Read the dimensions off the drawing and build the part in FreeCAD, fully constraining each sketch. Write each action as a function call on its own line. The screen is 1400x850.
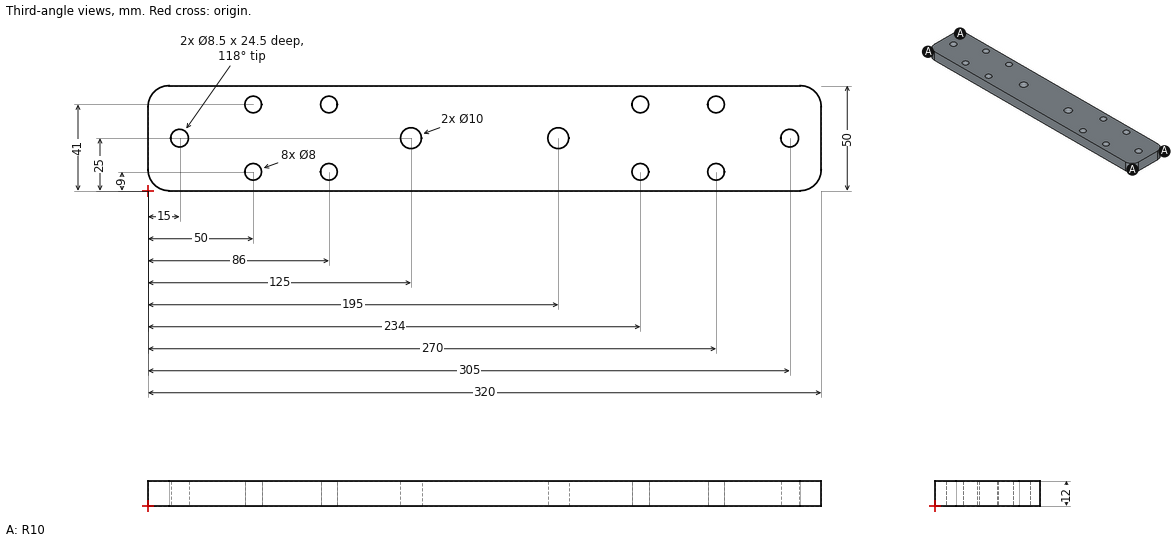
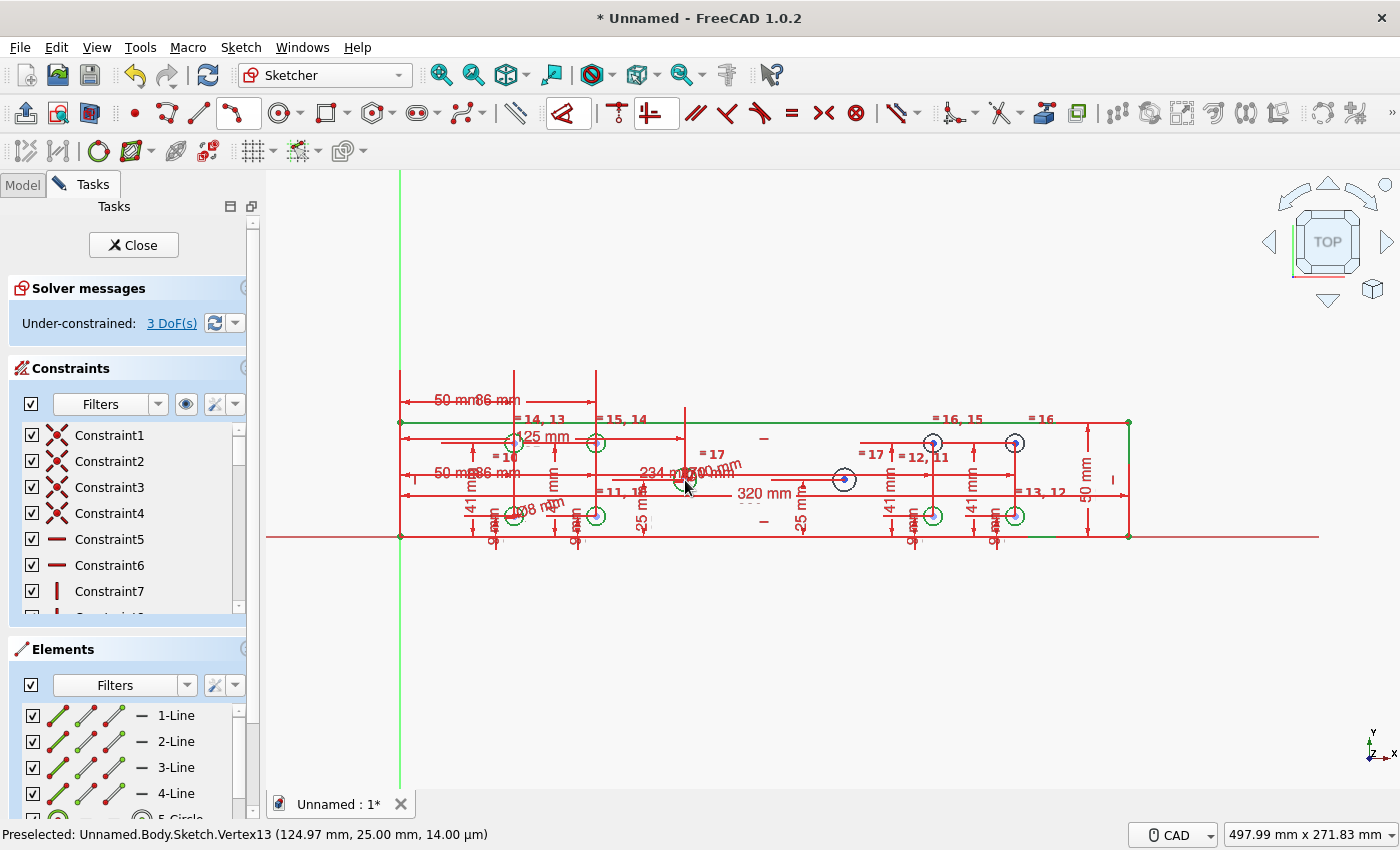
click(844, 480)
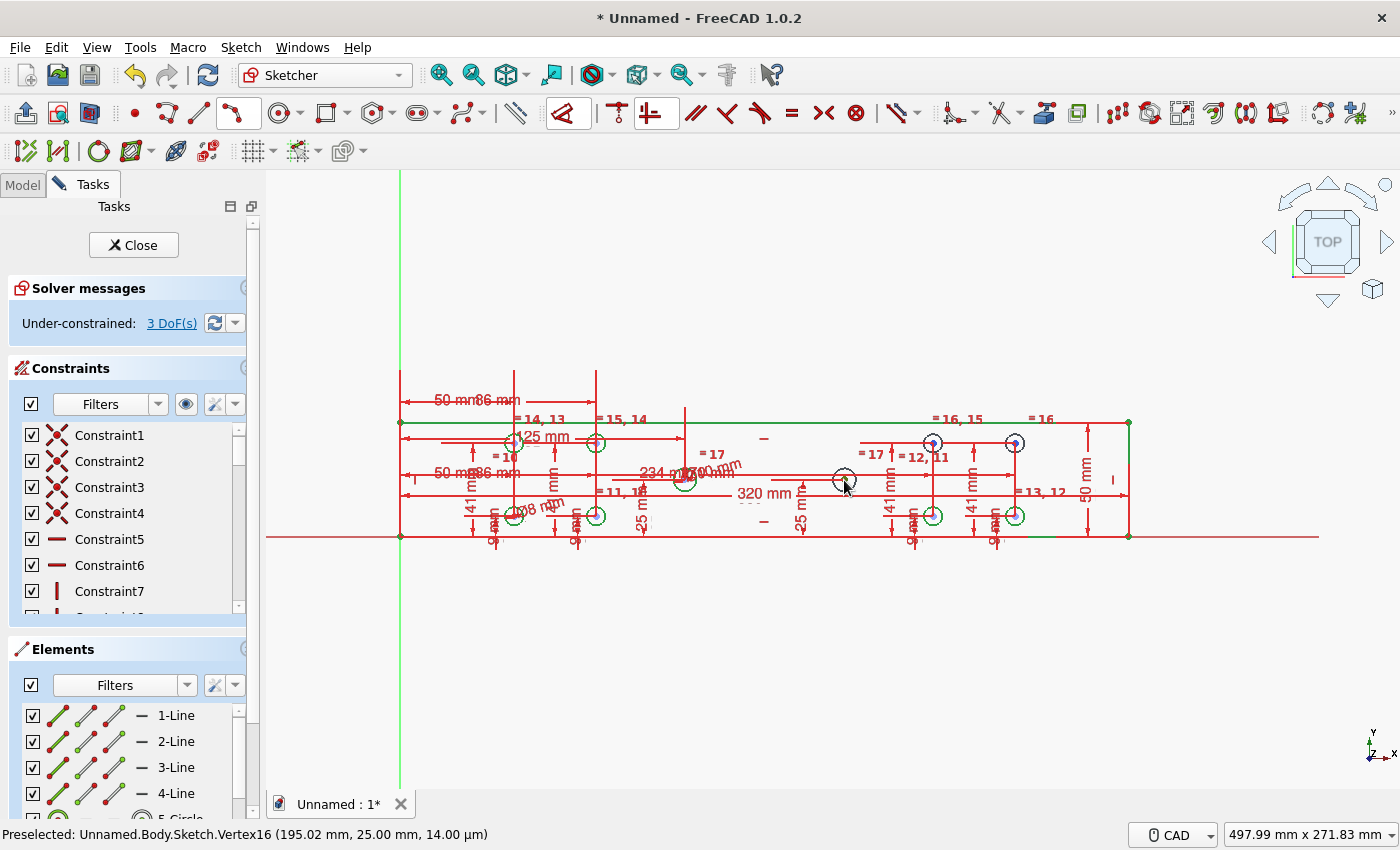
key(l)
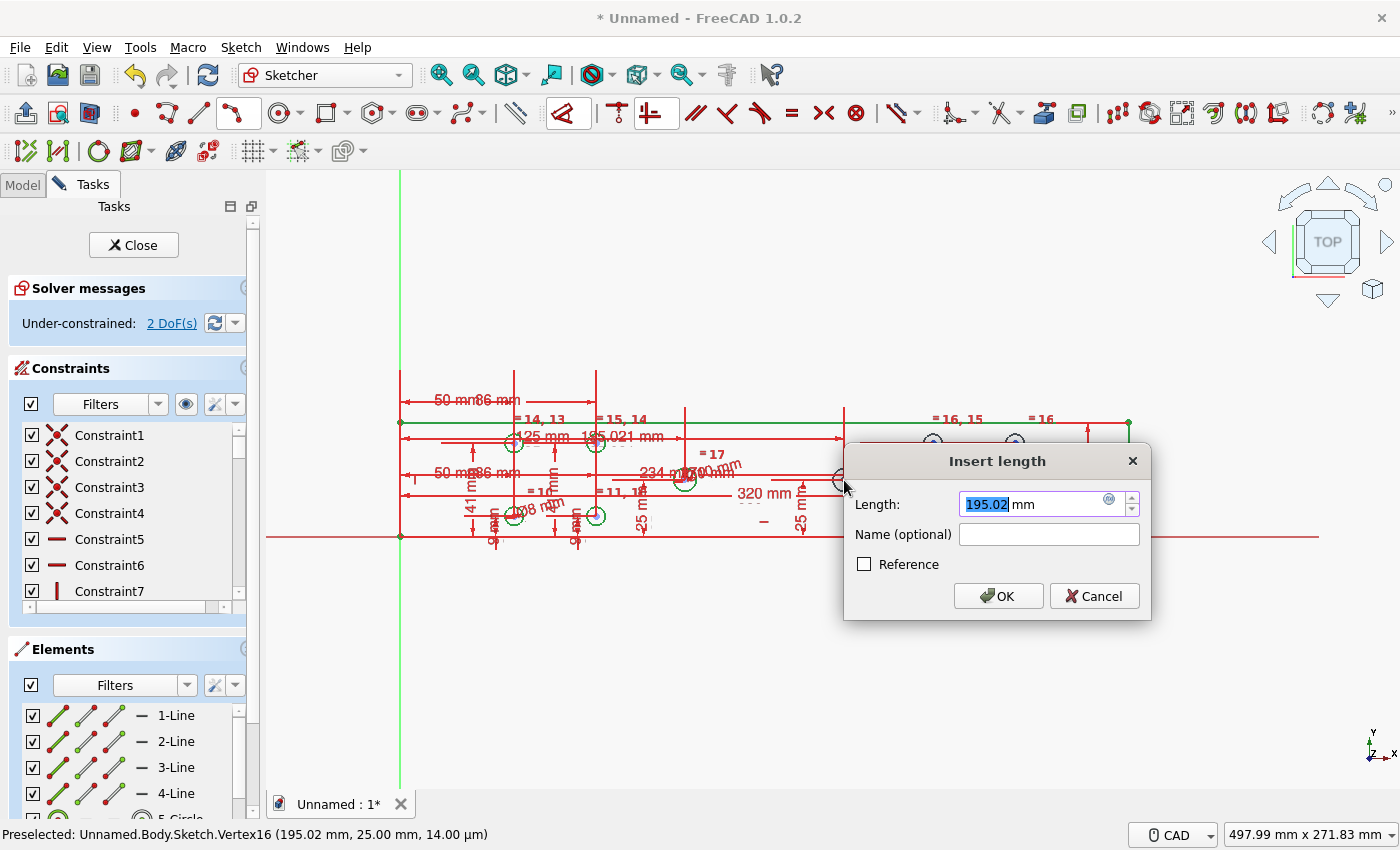
text(195)
key(Return)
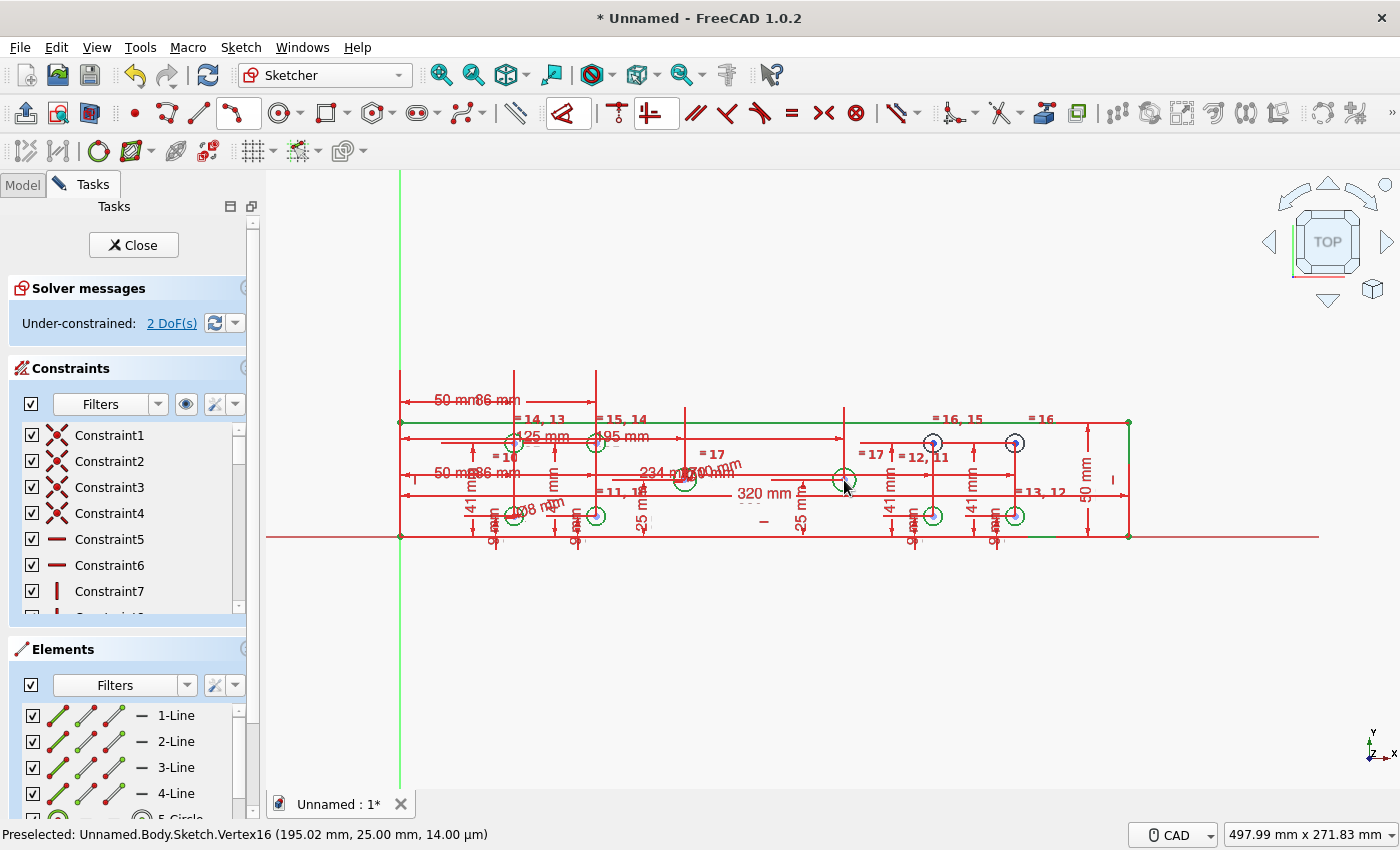
click(933, 443)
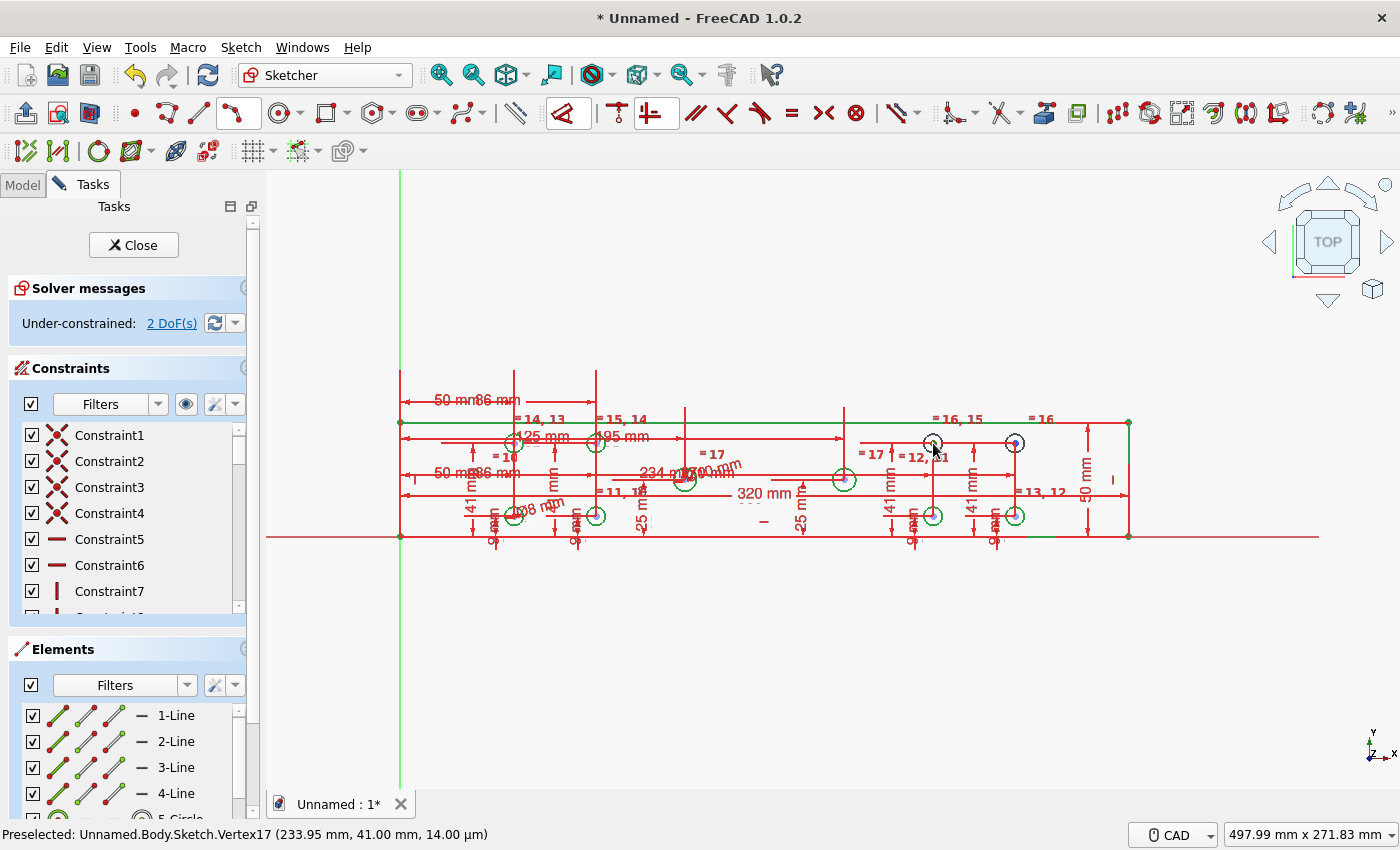
key(l)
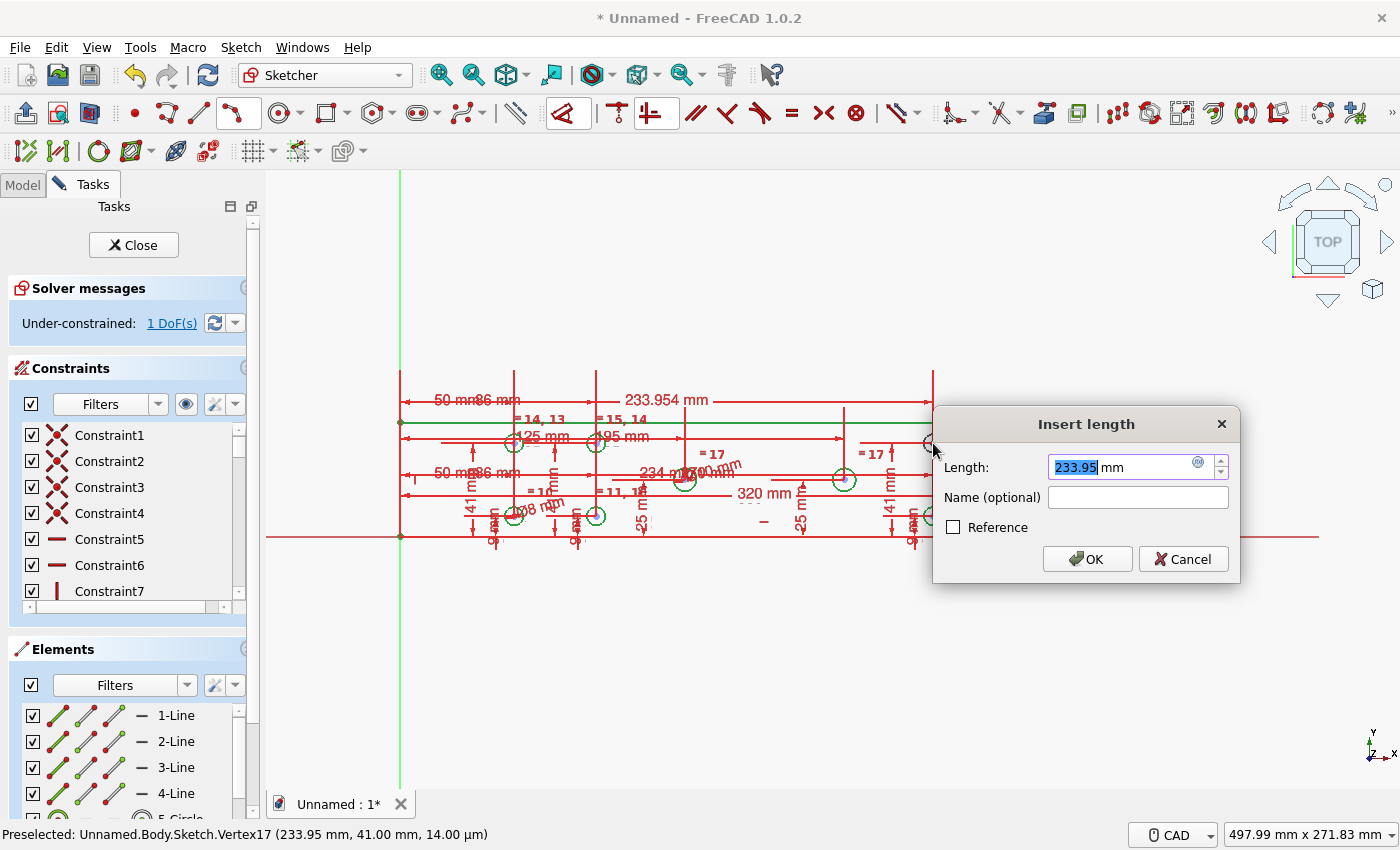
text(234)
key(Return)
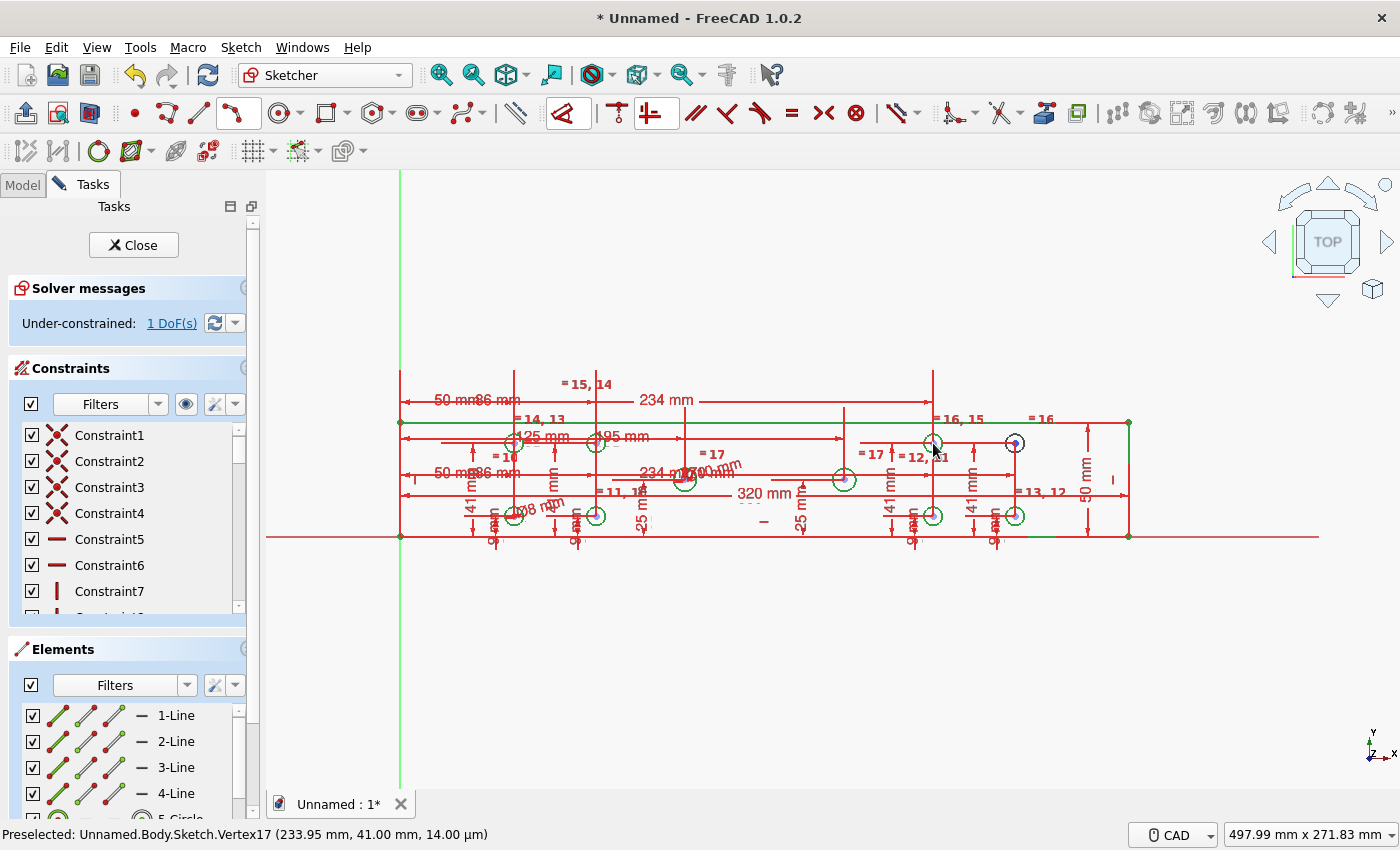
click(1015, 443)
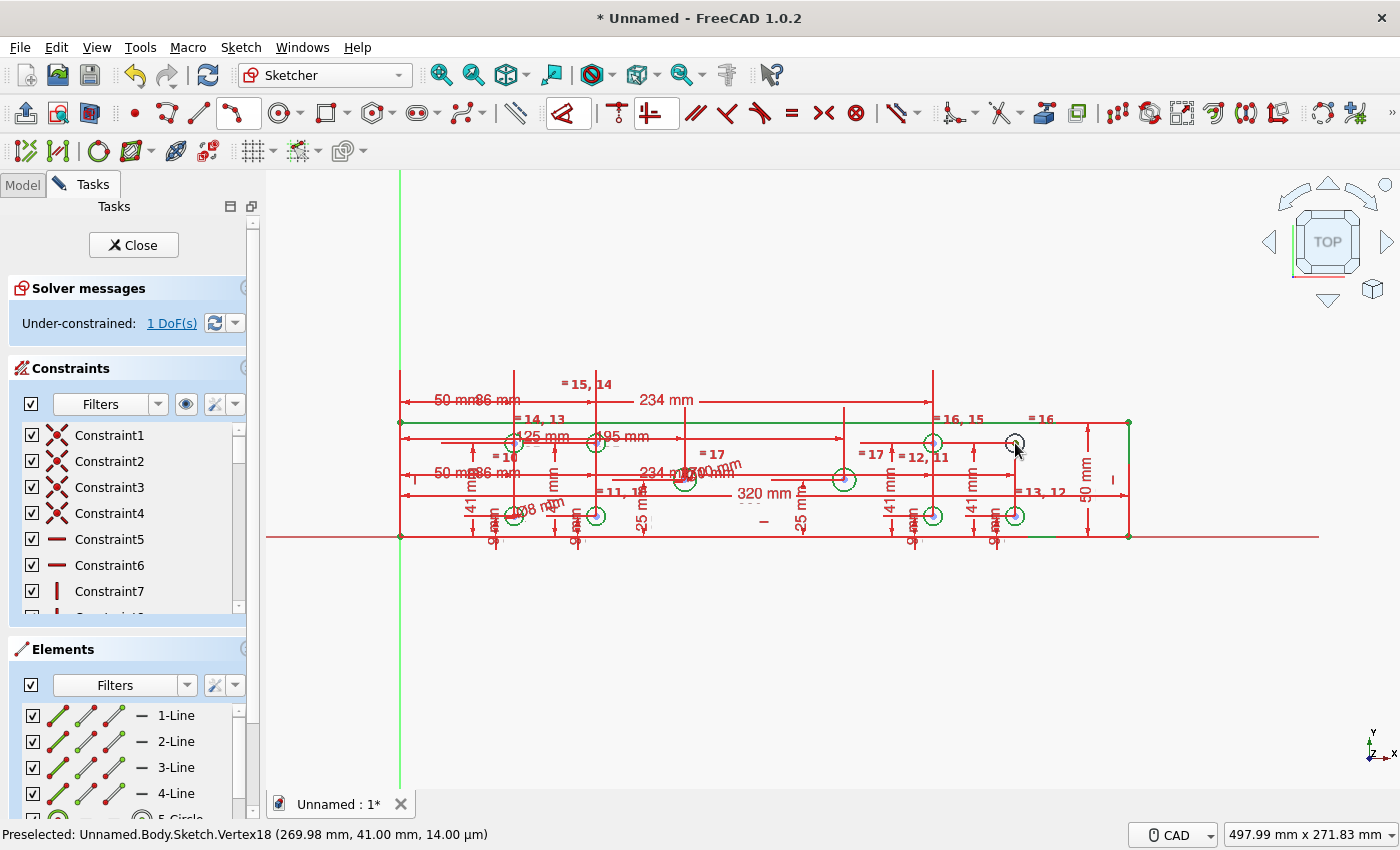
key(l)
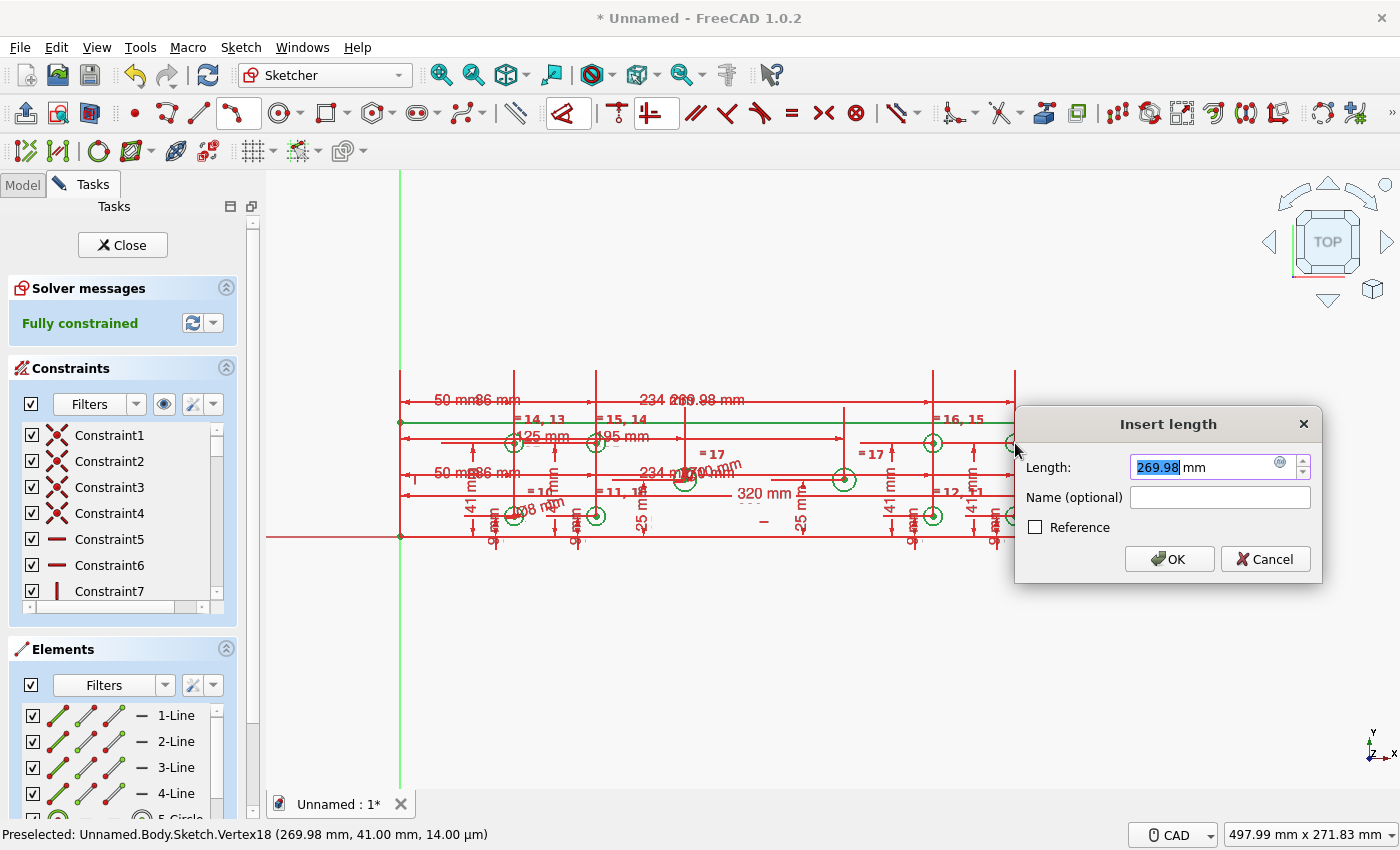
text(270)
key(Return)